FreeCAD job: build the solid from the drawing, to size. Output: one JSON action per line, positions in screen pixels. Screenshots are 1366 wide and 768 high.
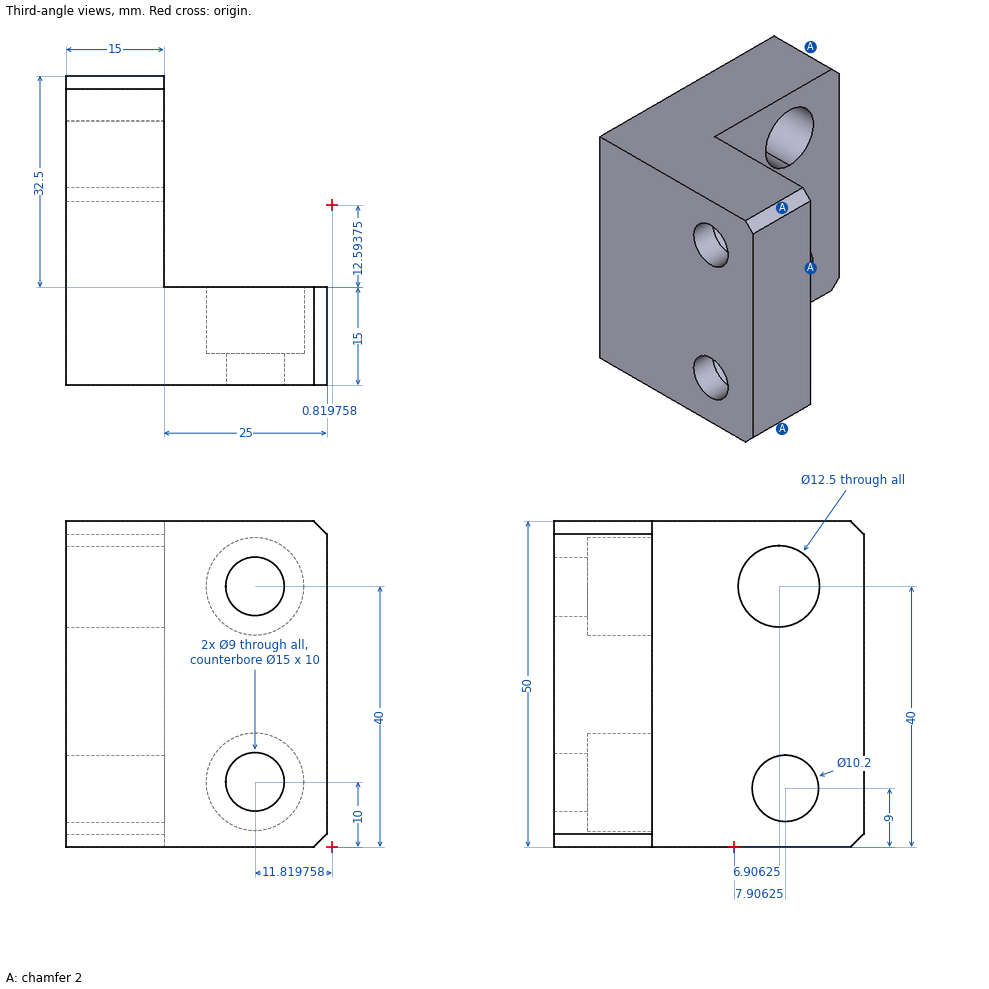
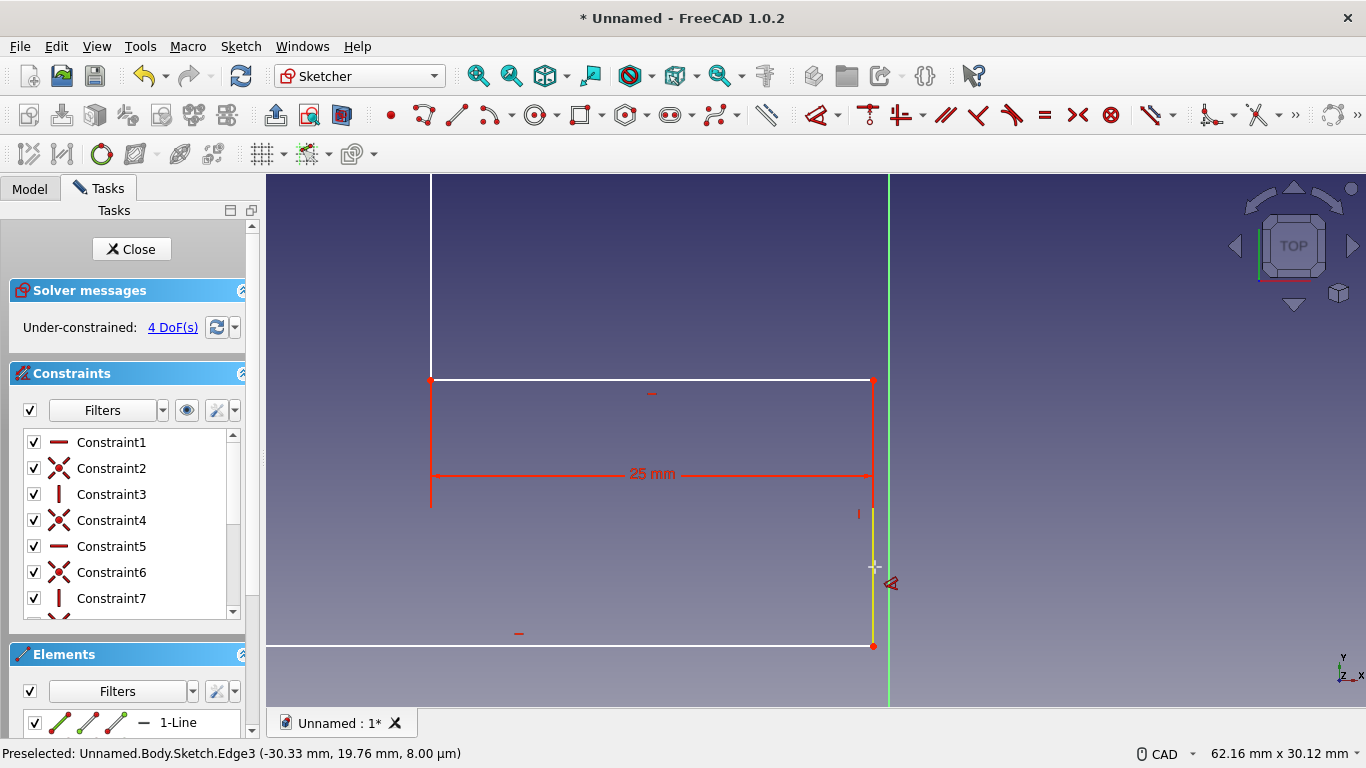
{"action": "left_click", "coordinate": [873, 567]}
{"action": "left_click", "coordinate": [907, 513]}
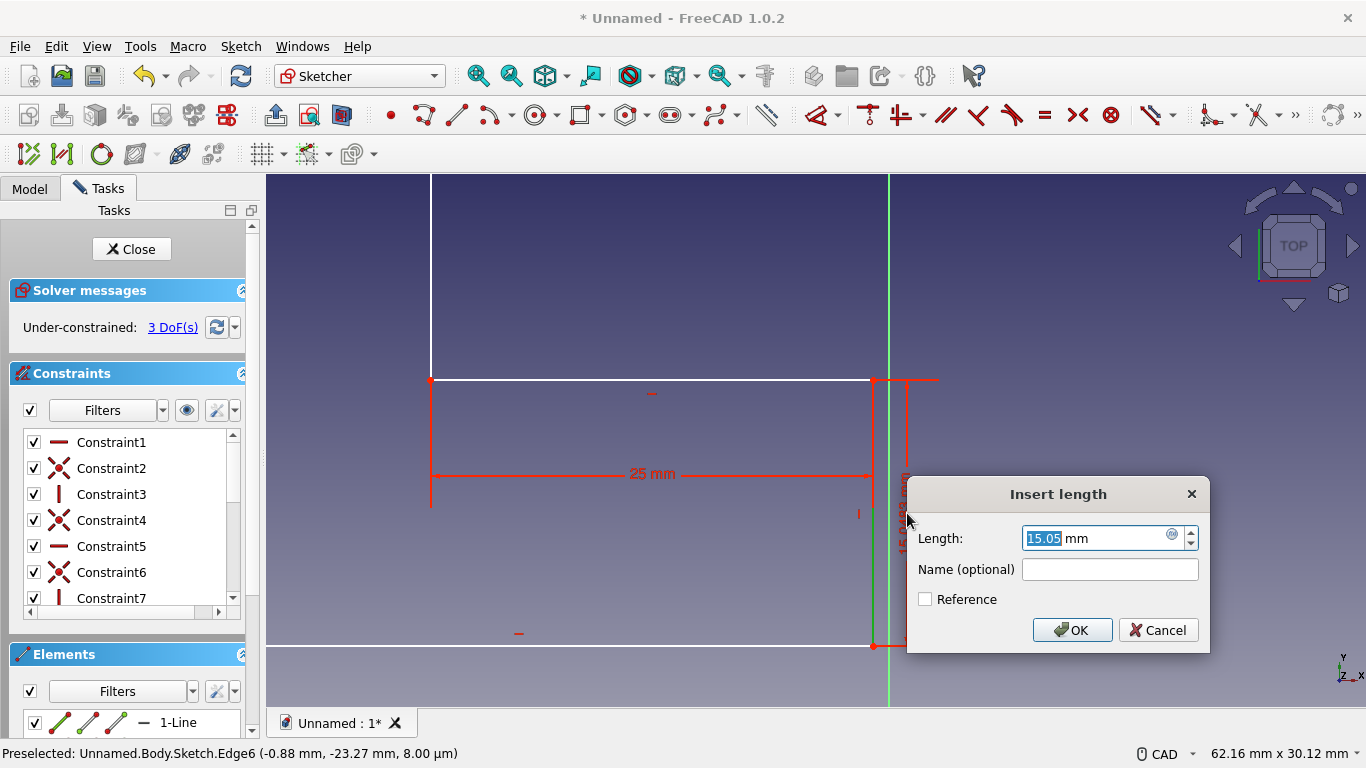
{"action": "type", "text": "15"}
{"action": "key", "text": "Return"}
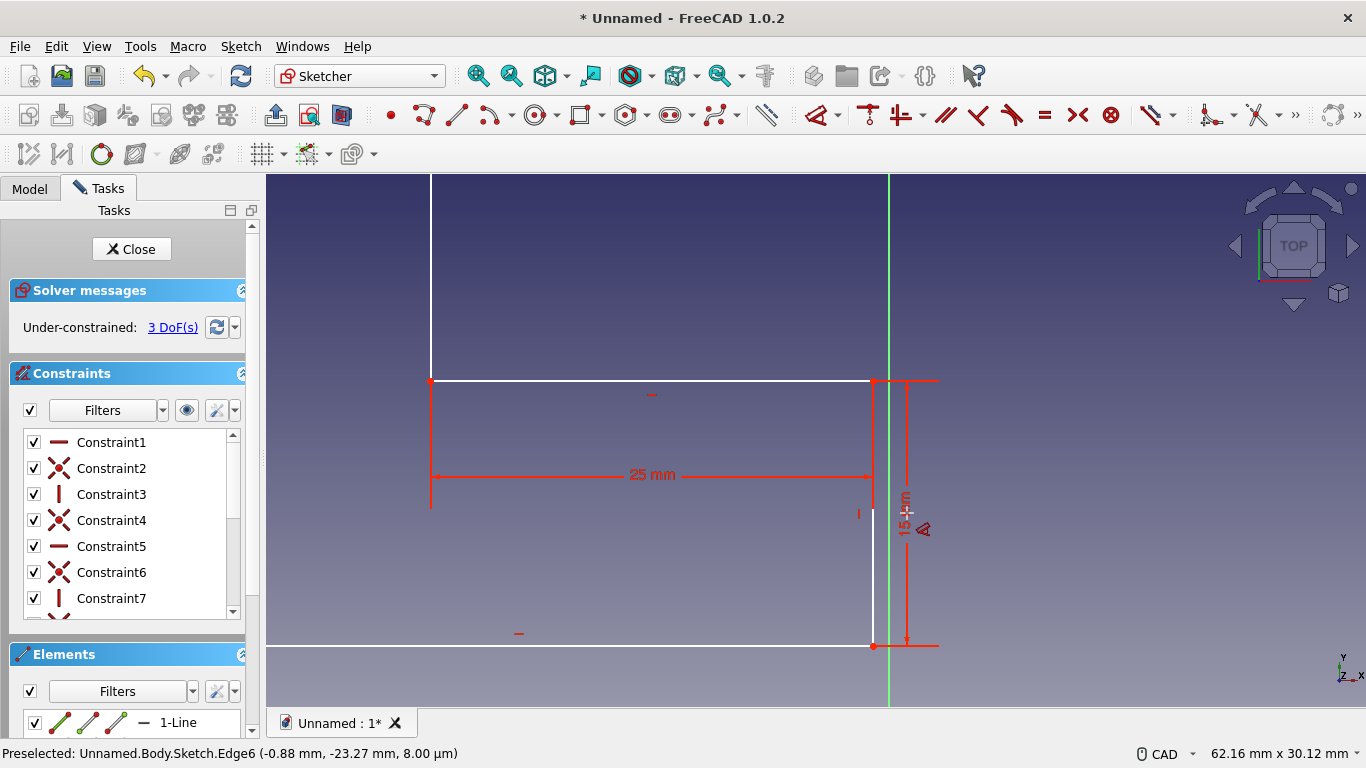
{"action": "left_click", "coordinate": [431, 209]}
{"action": "left_click", "coordinate": [397, 292]}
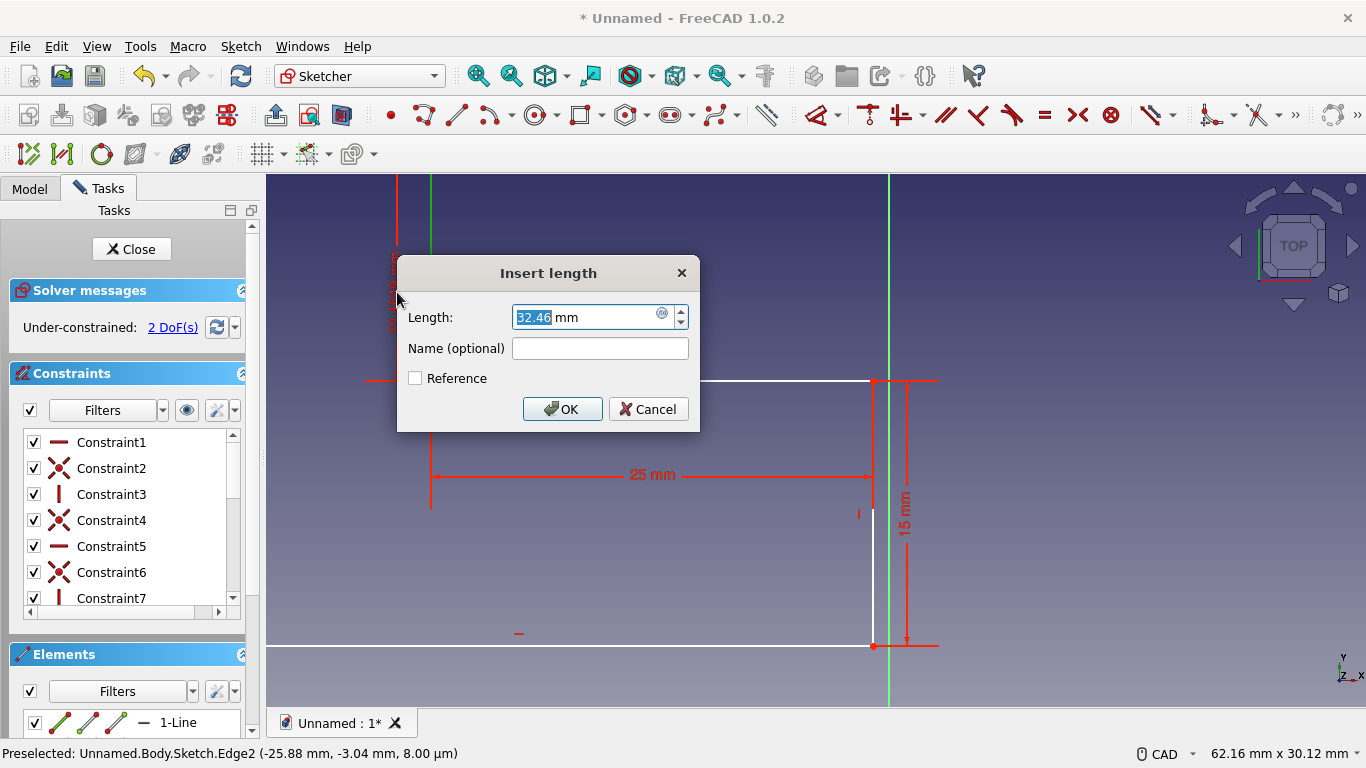
{"action": "type", "text": "32.5"}
{"action": "key", "text": "Return"}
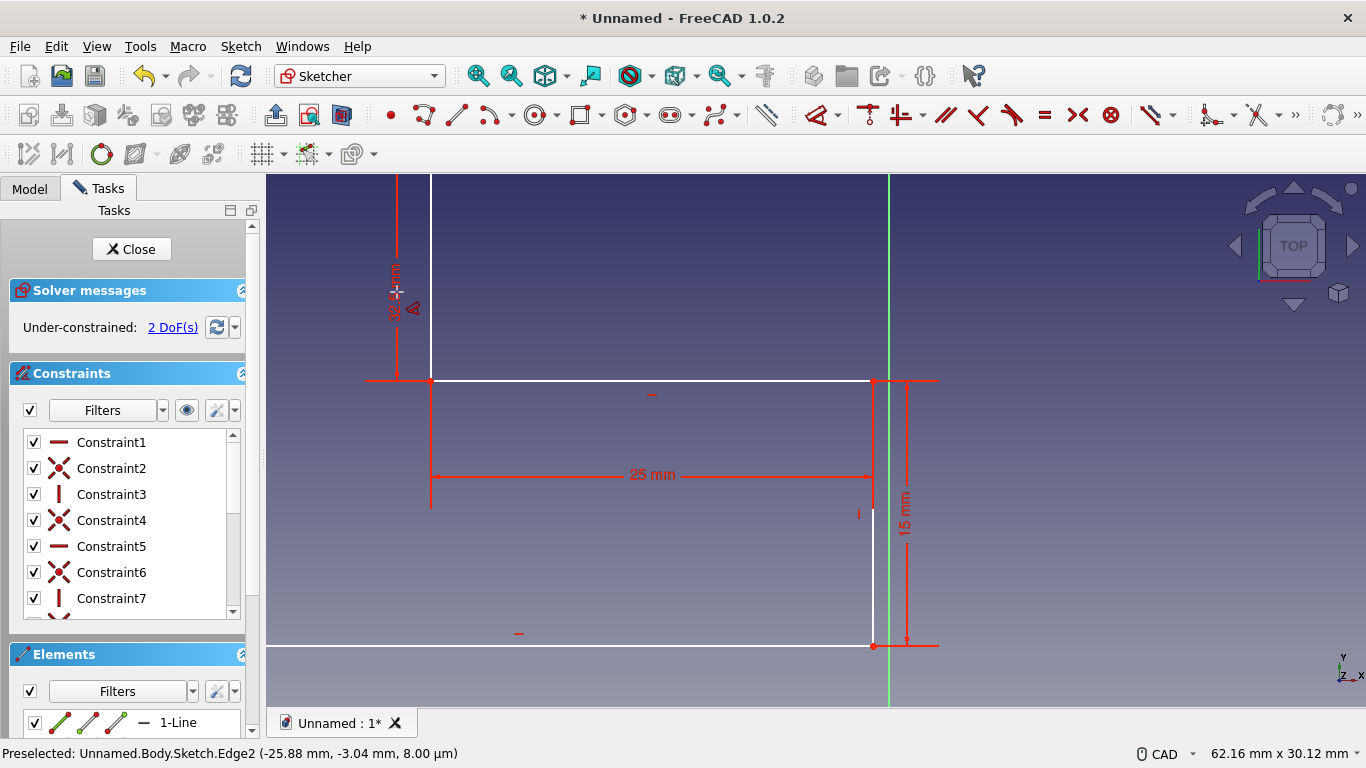
{"action": "scroll", "coordinate": [873, 381], "scroll_direction": "up", "scroll_amount": 6}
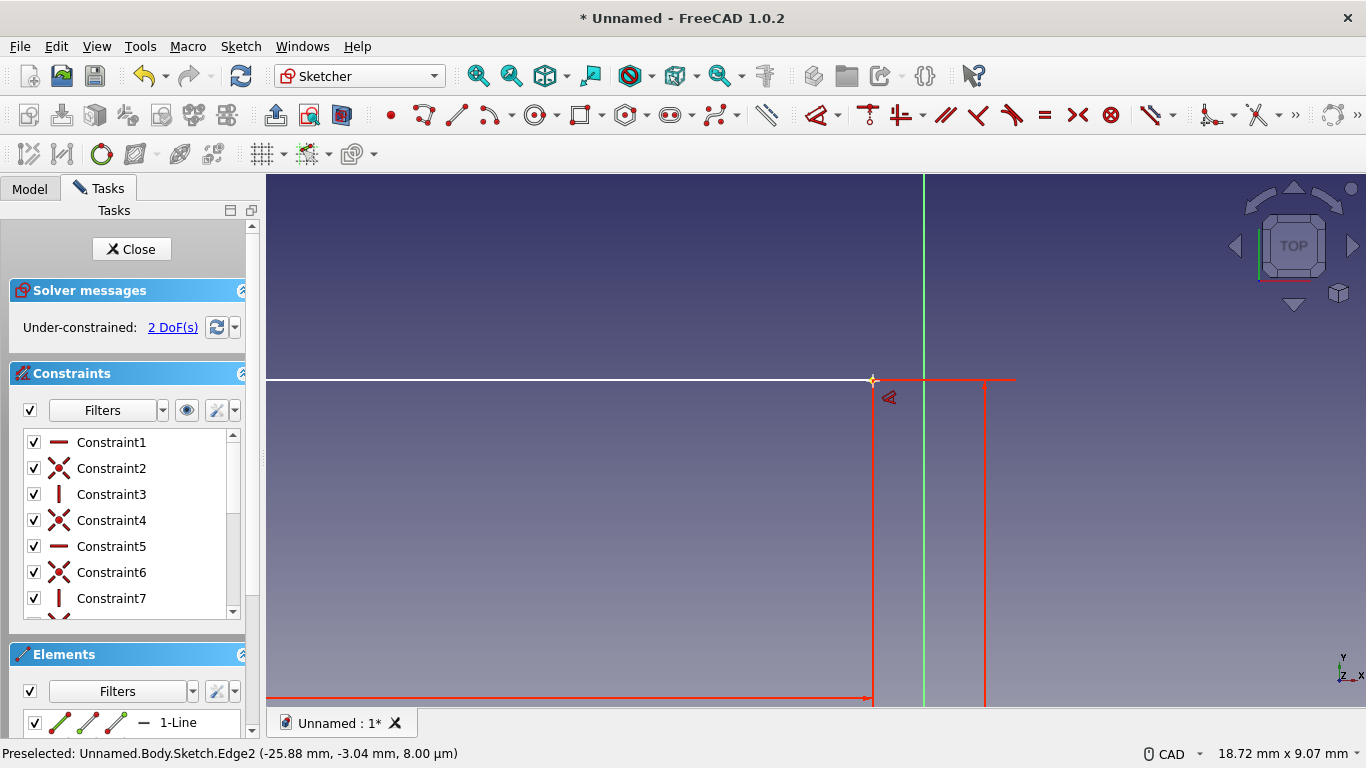
{"action": "left_click", "coordinate": [873, 380]}
{"action": "left_click", "coordinate": [898, 414]}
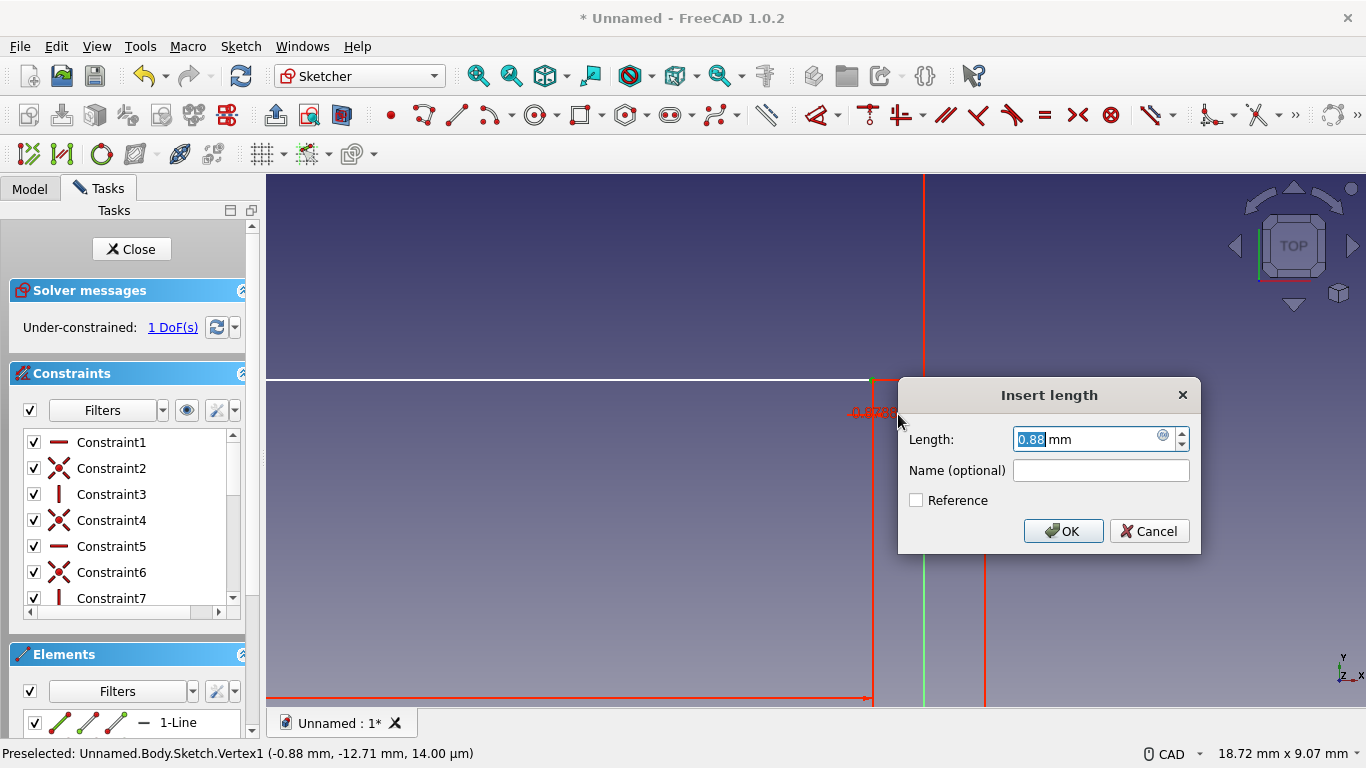
{"action": "type", "text": "0.819758"}
{"action": "key", "text": "Return"}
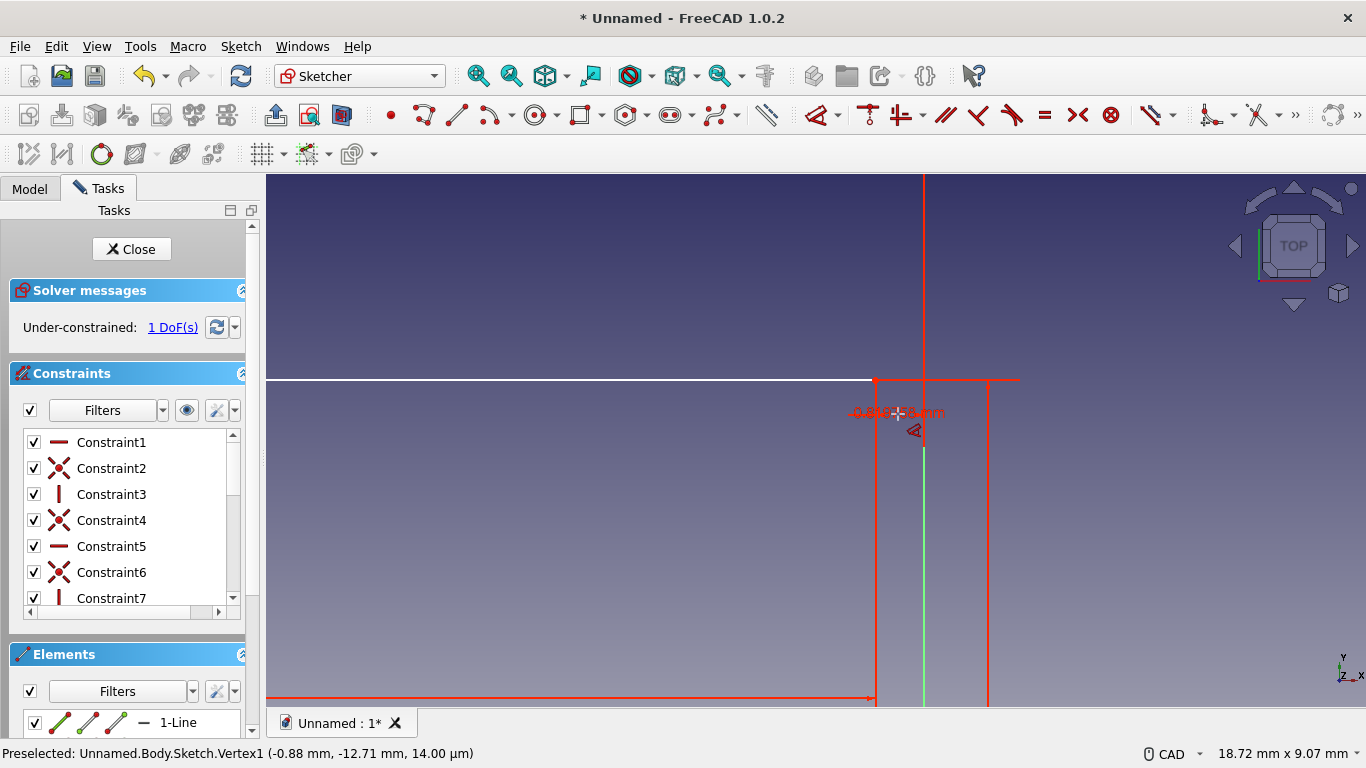
{"action": "scroll", "coordinate": [875, 513], "scroll_direction": "down", "scroll_amount": 11}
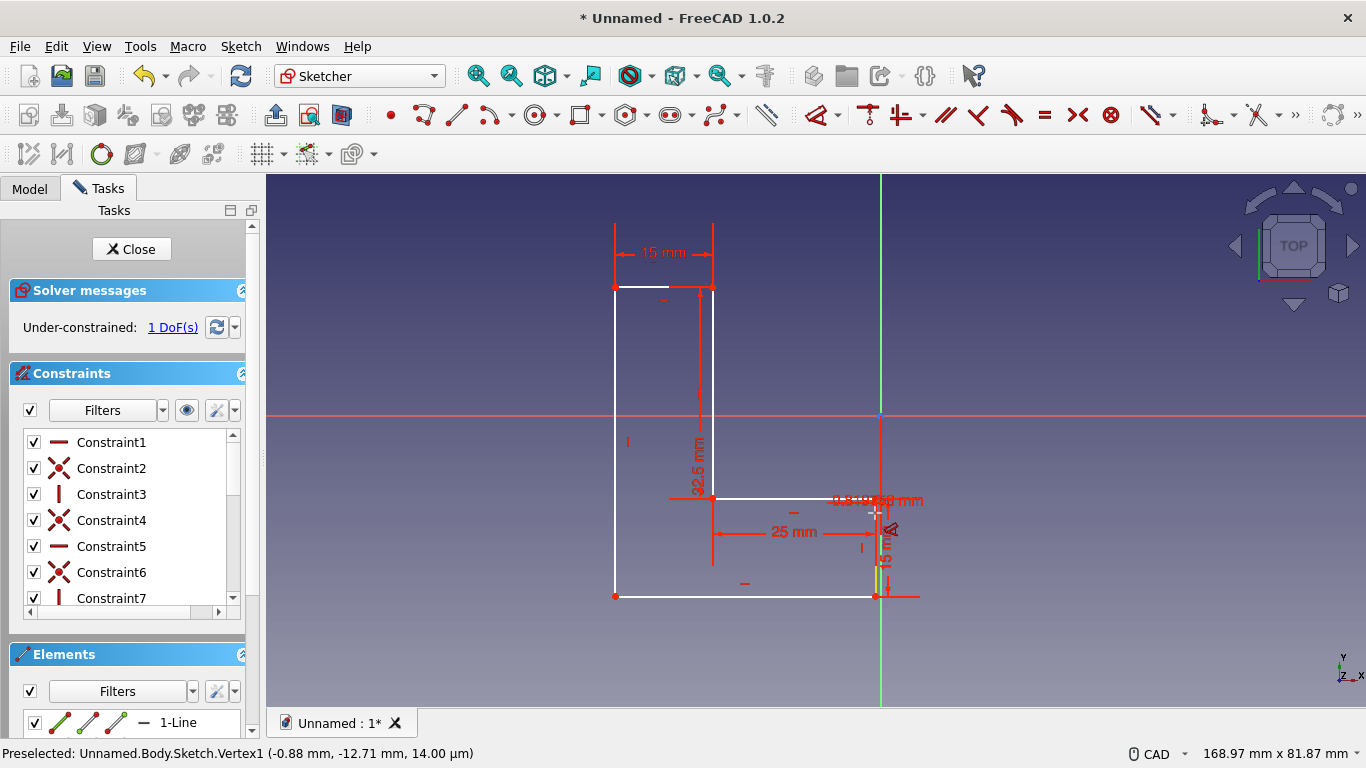
{"action": "left_click", "coordinate": [876, 499]}
{"action": "left_click", "coordinate": [915, 457]}